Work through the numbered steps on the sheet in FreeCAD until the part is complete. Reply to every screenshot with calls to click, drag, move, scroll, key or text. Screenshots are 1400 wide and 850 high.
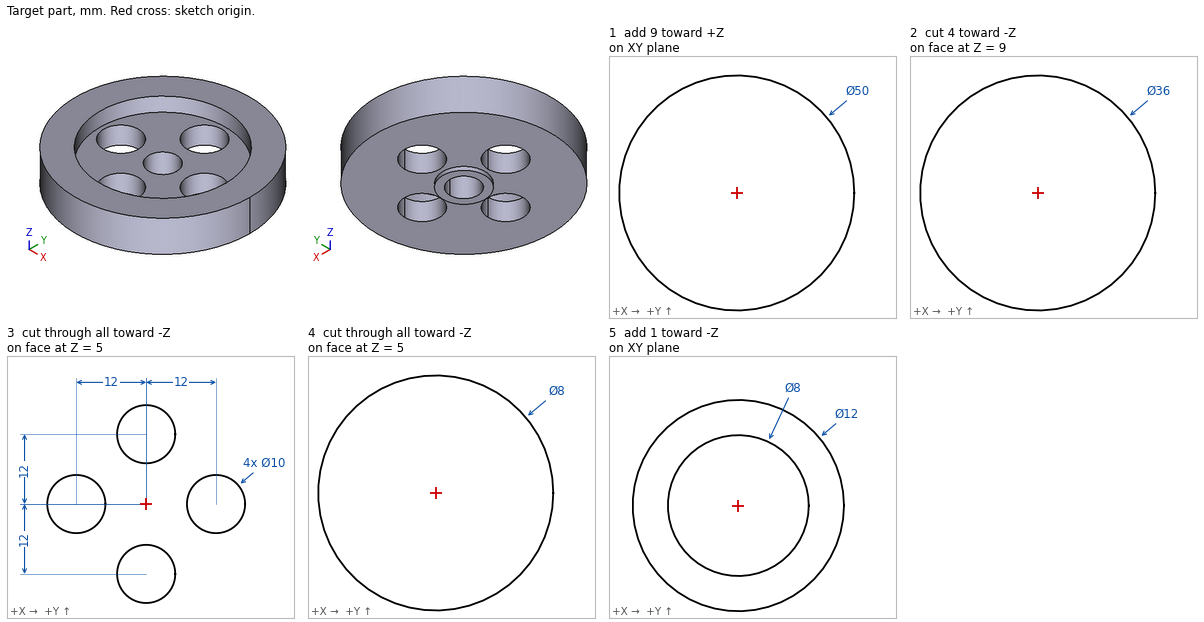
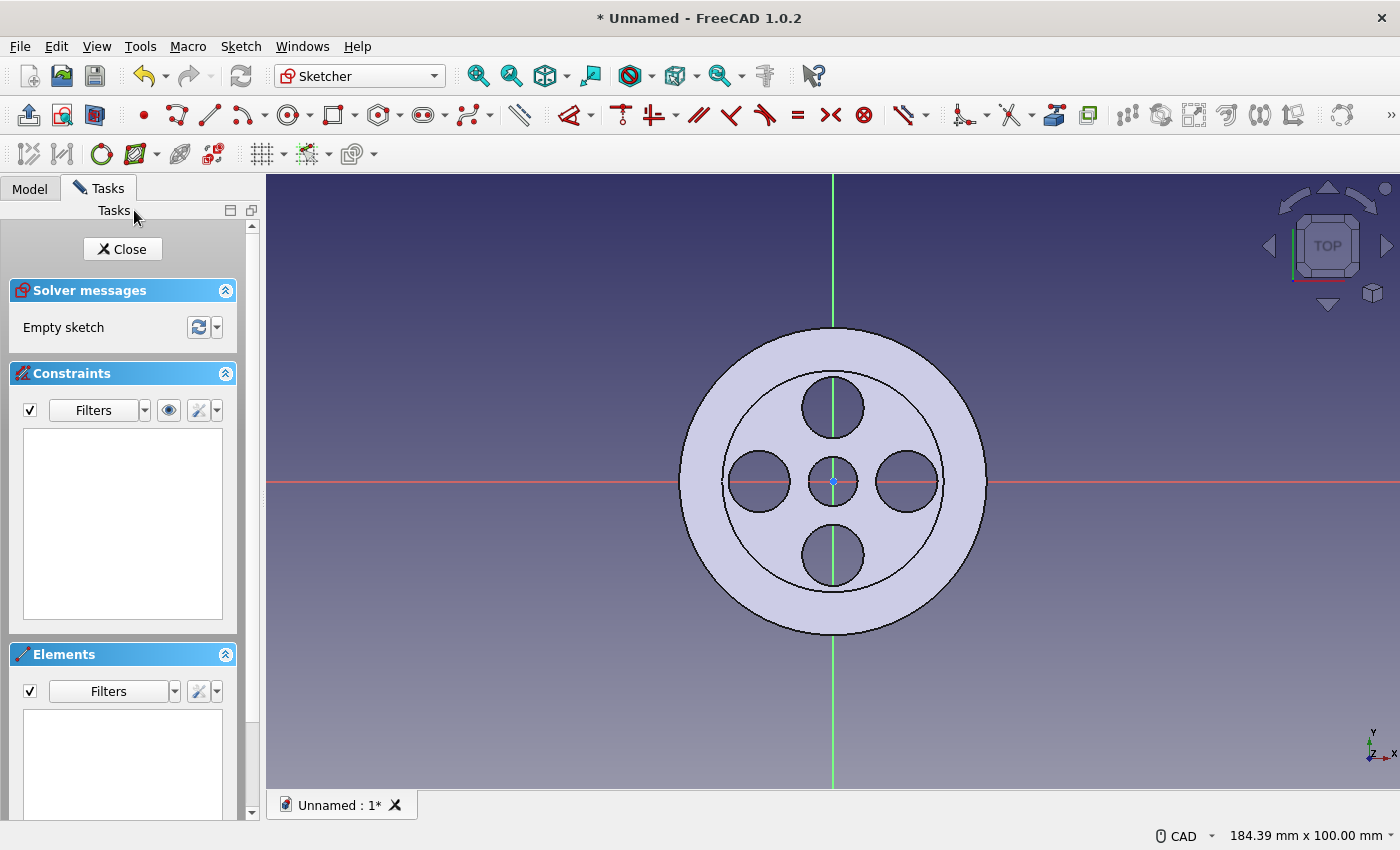
click(95, 116)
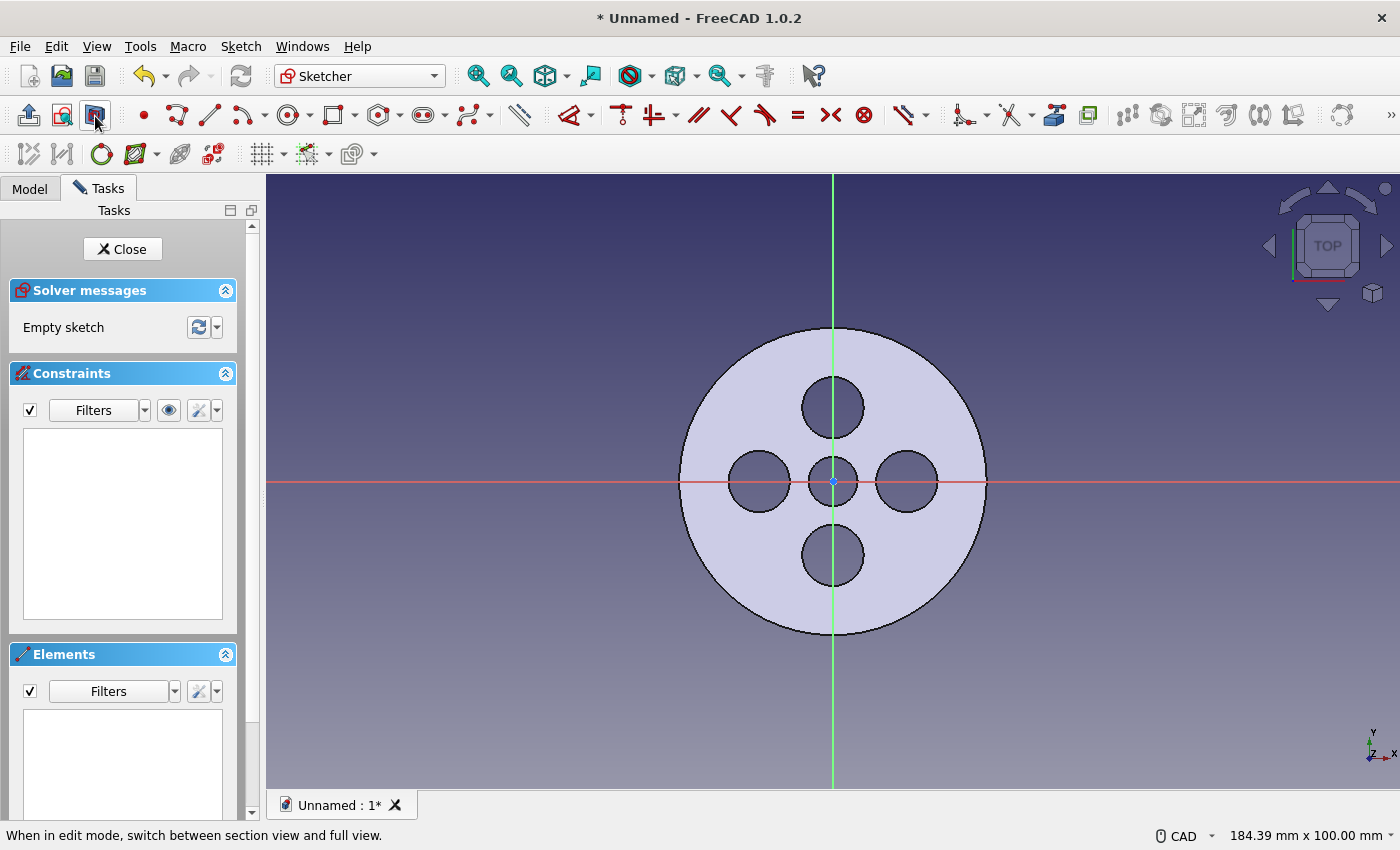
scroll(850, 482, up, 8)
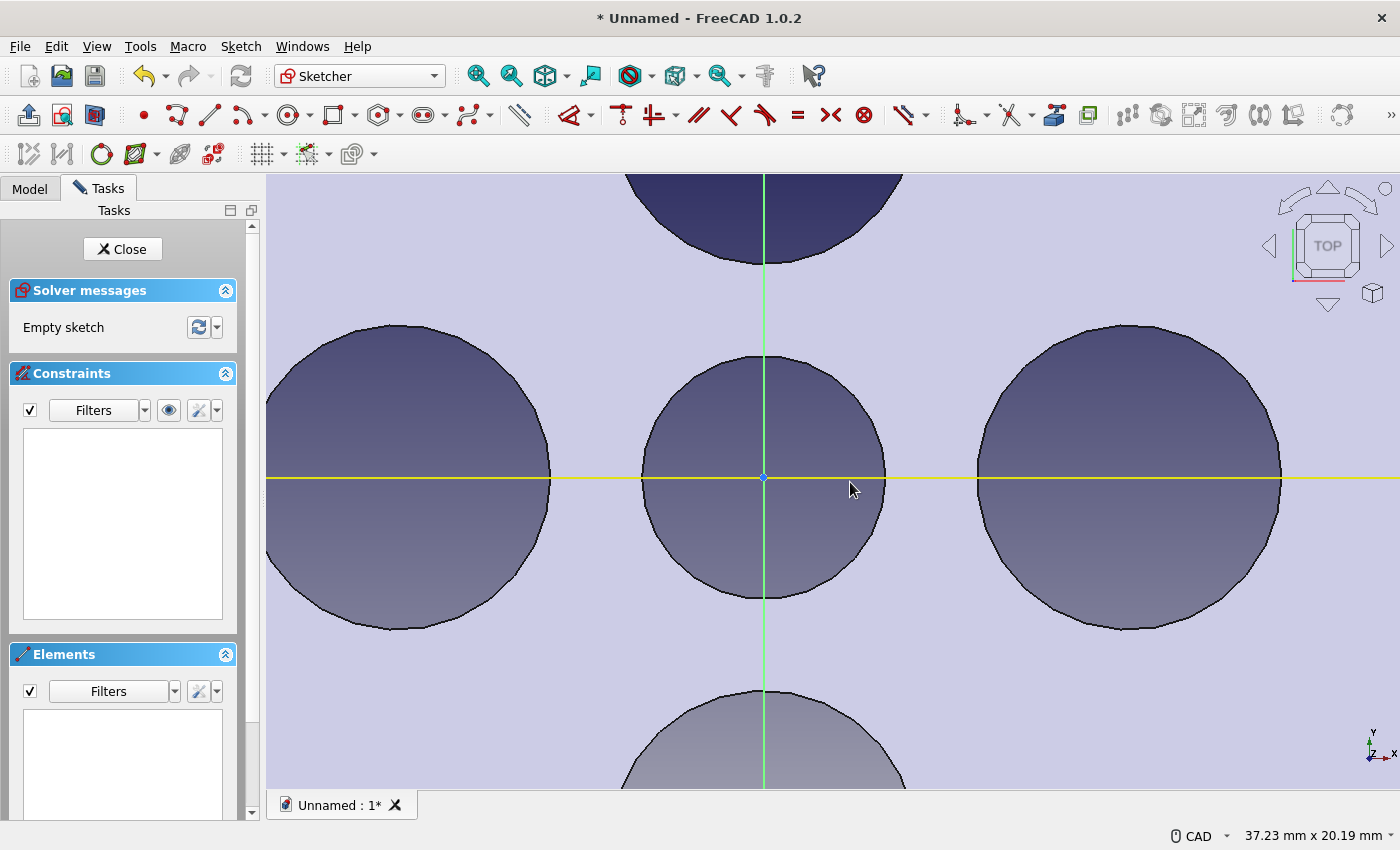
click(288, 116)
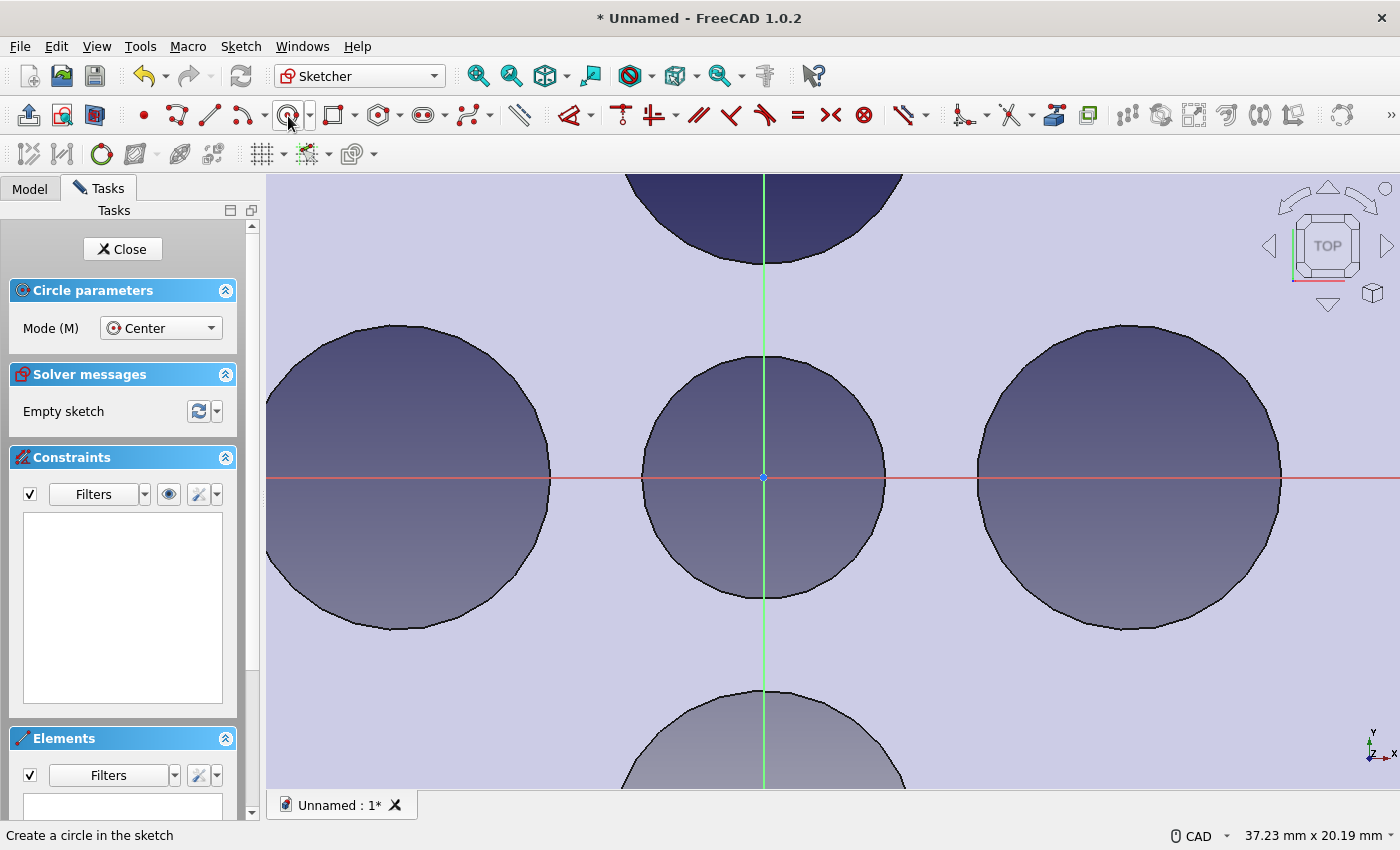
click(764, 478)
move(893, 348)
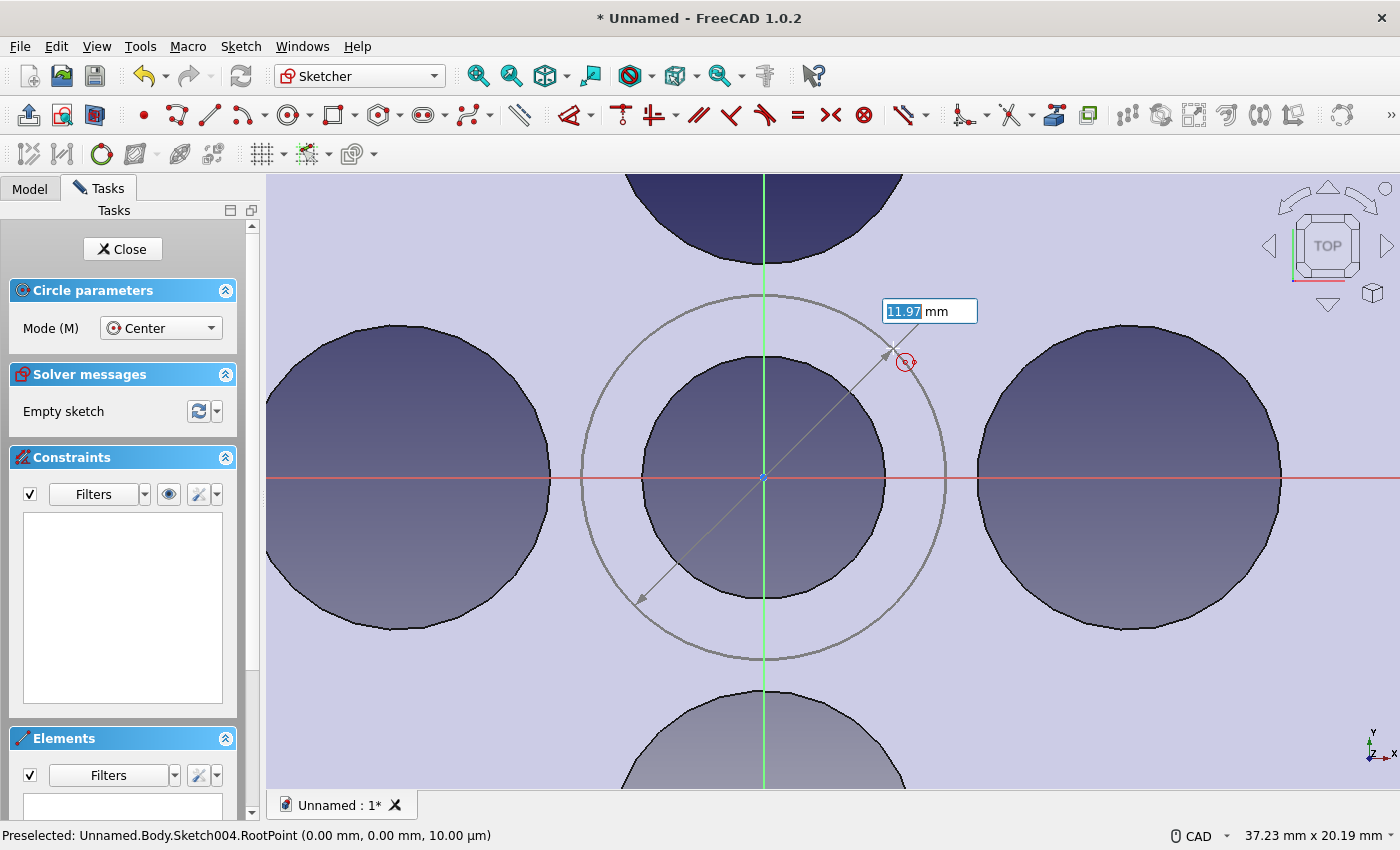
text(12)
key(Return)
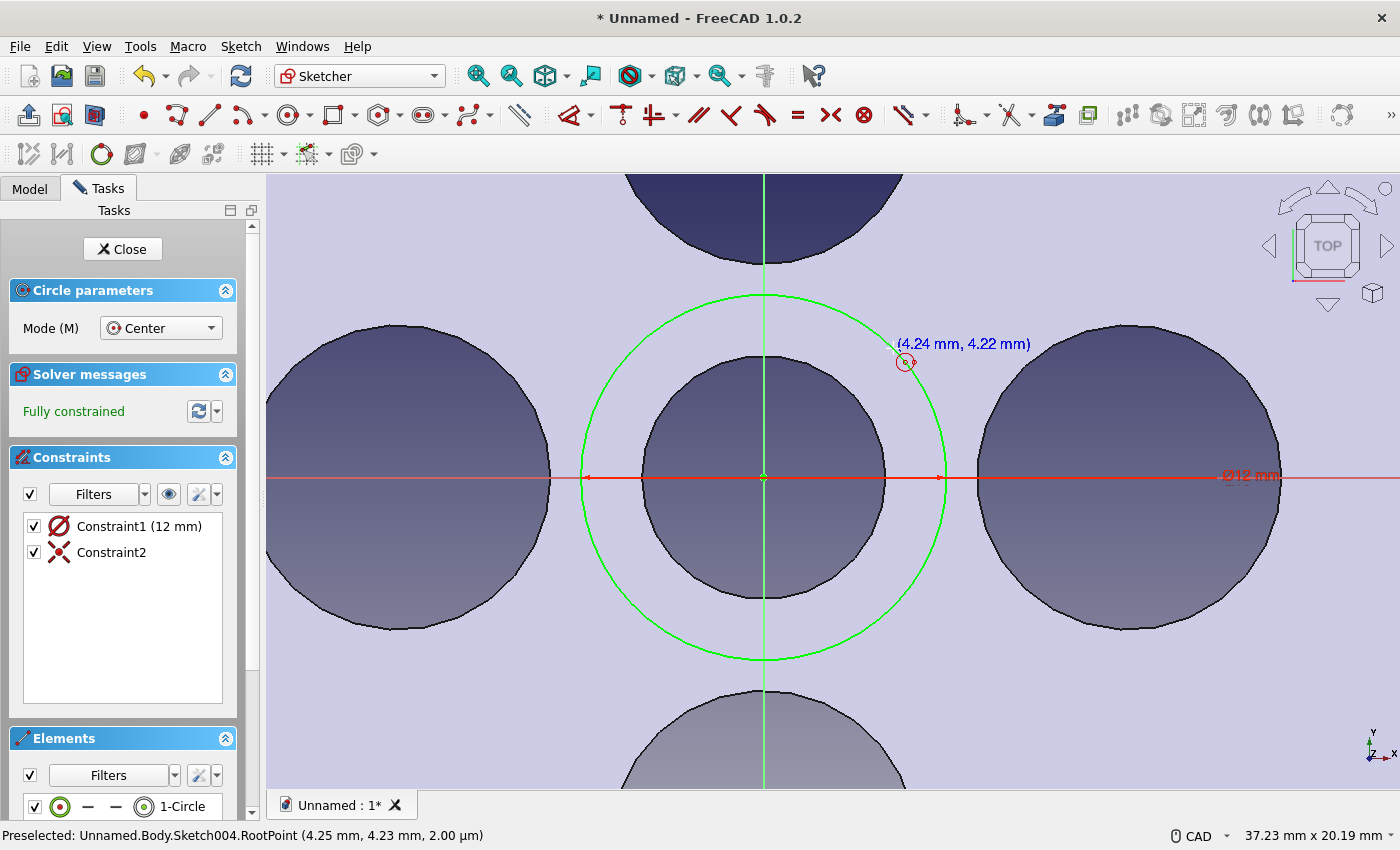
click(764, 478)
move(850, 391)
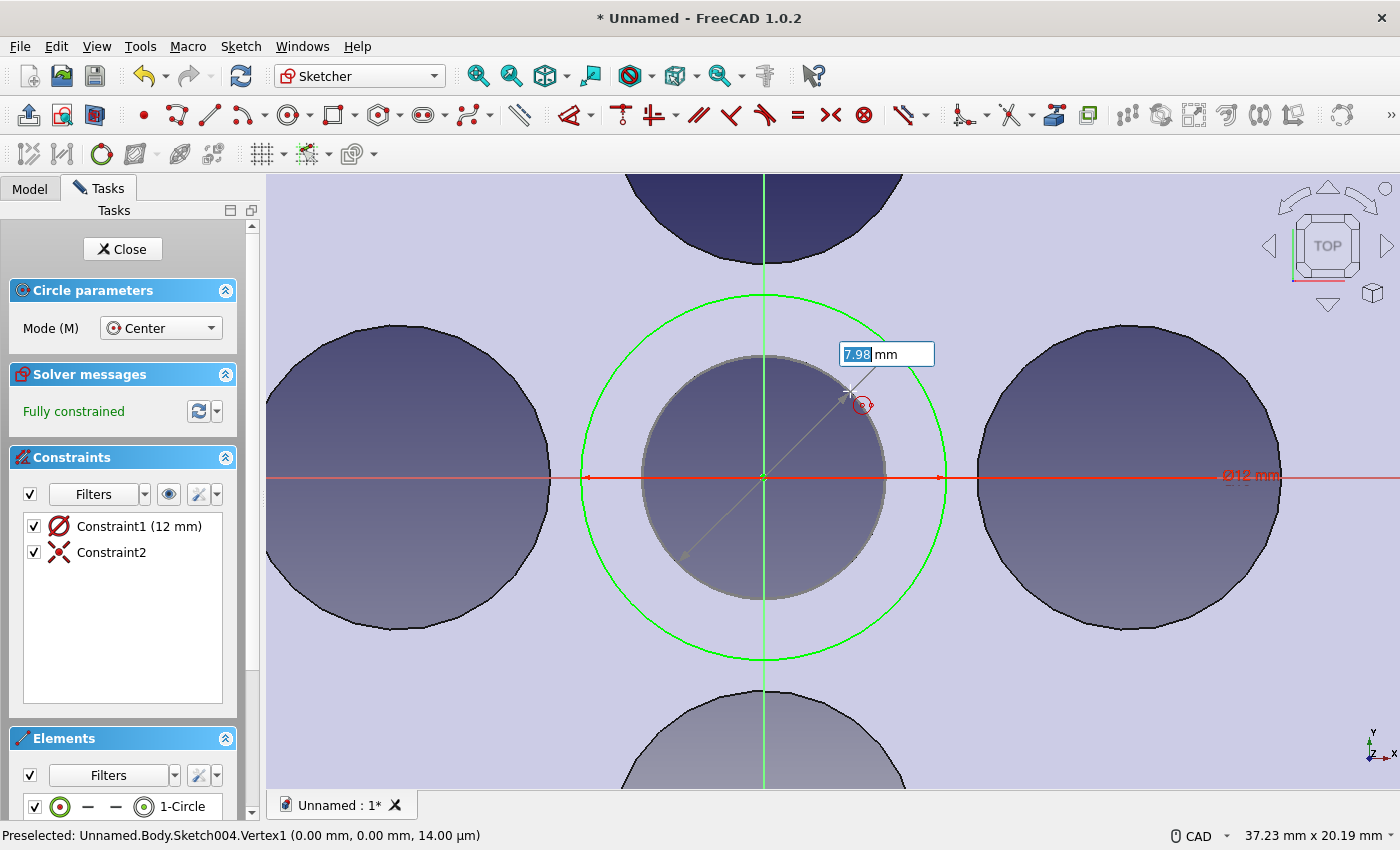
text(8)
key(Return)
key(Escape)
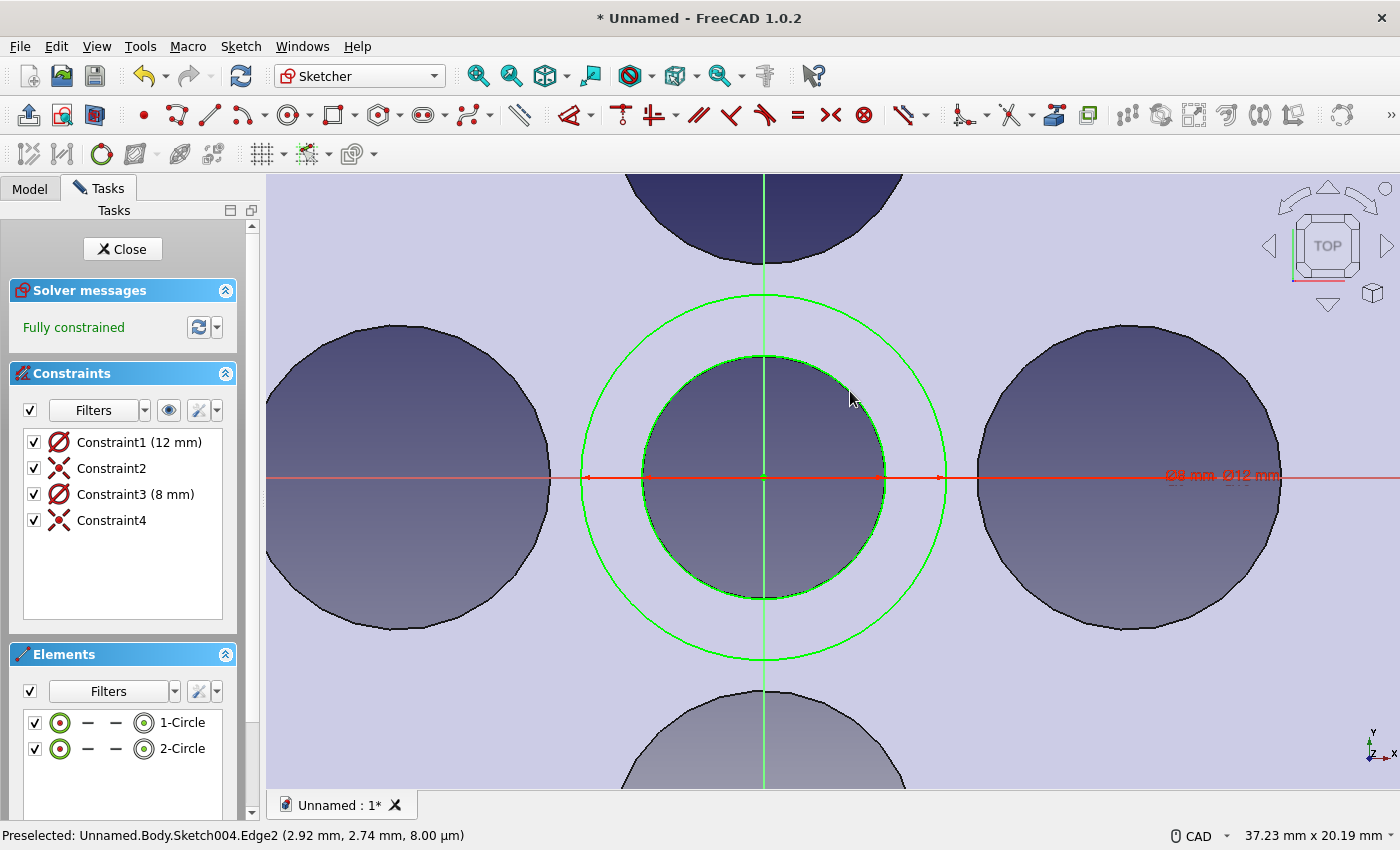
click(123, 249)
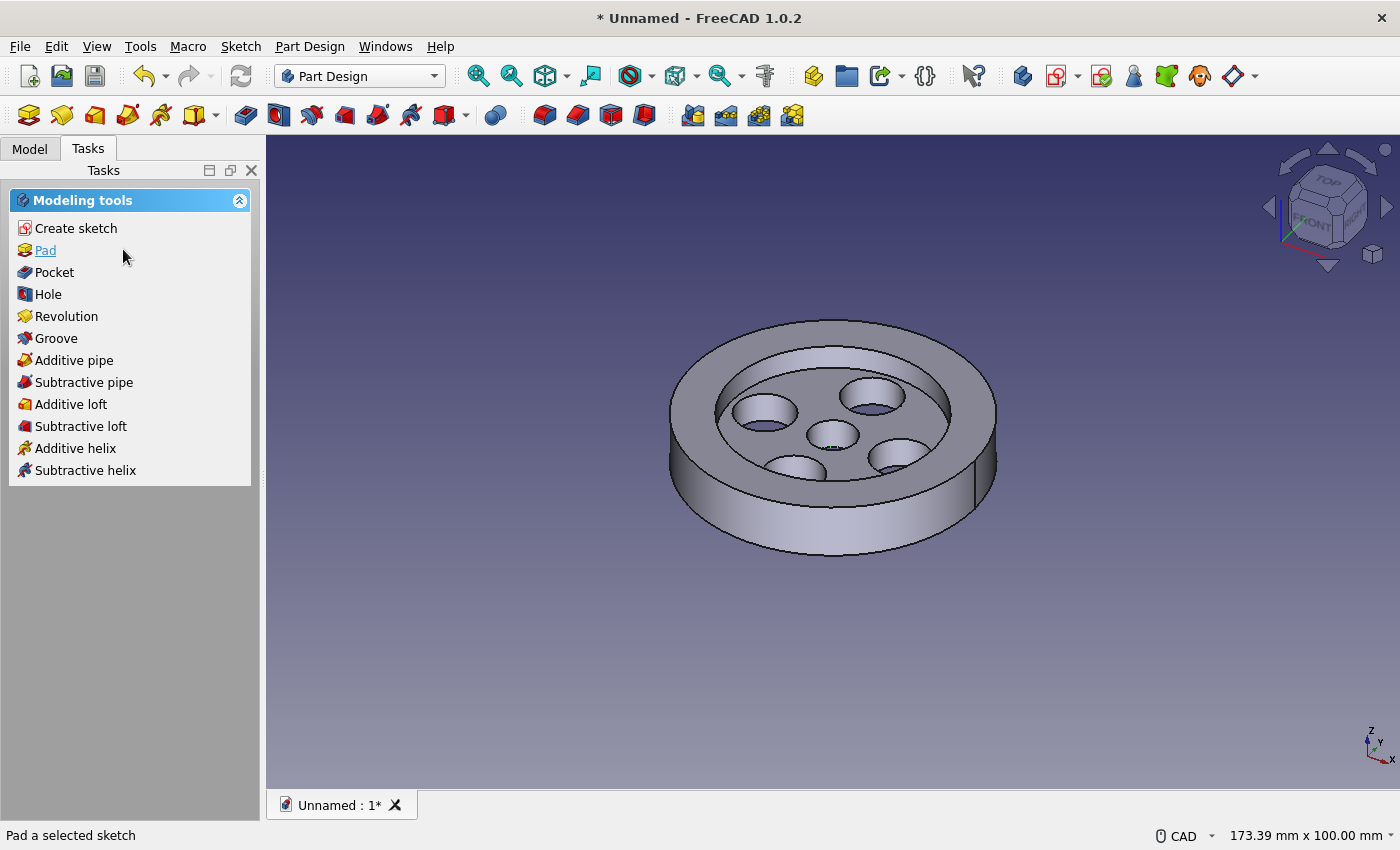
click(29, 116)